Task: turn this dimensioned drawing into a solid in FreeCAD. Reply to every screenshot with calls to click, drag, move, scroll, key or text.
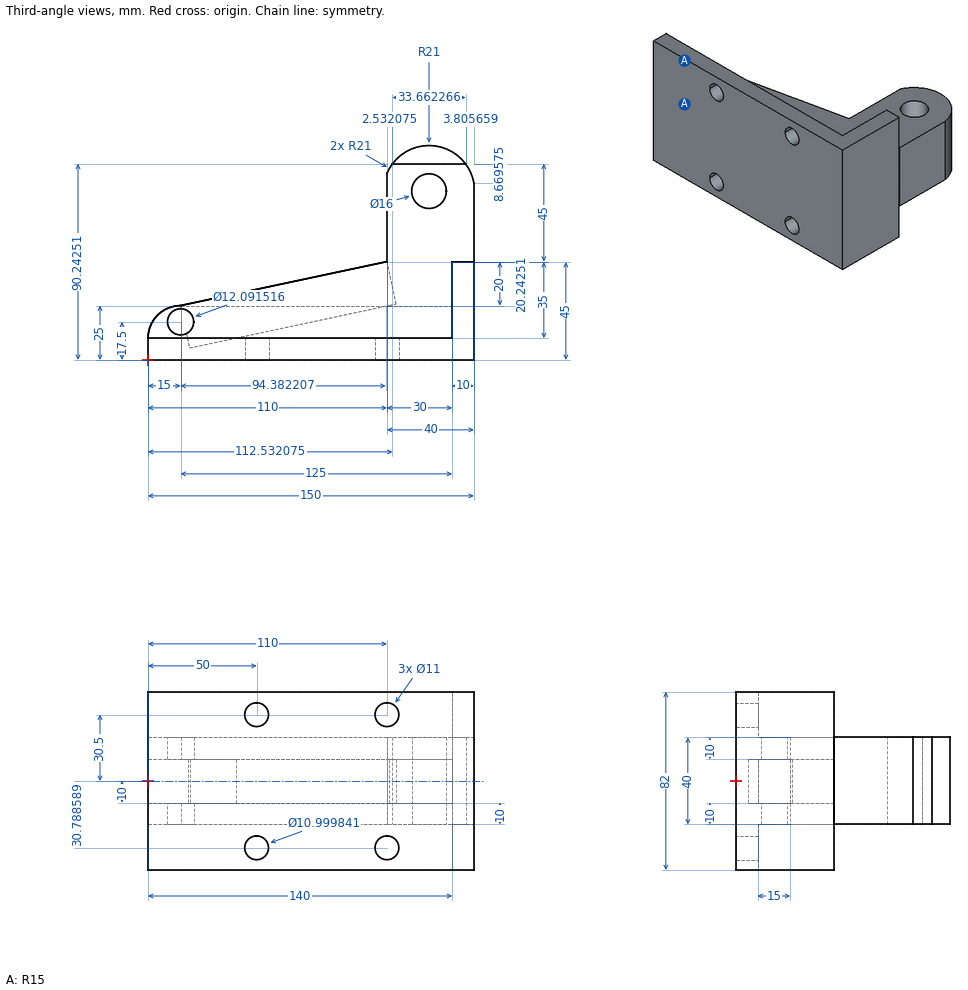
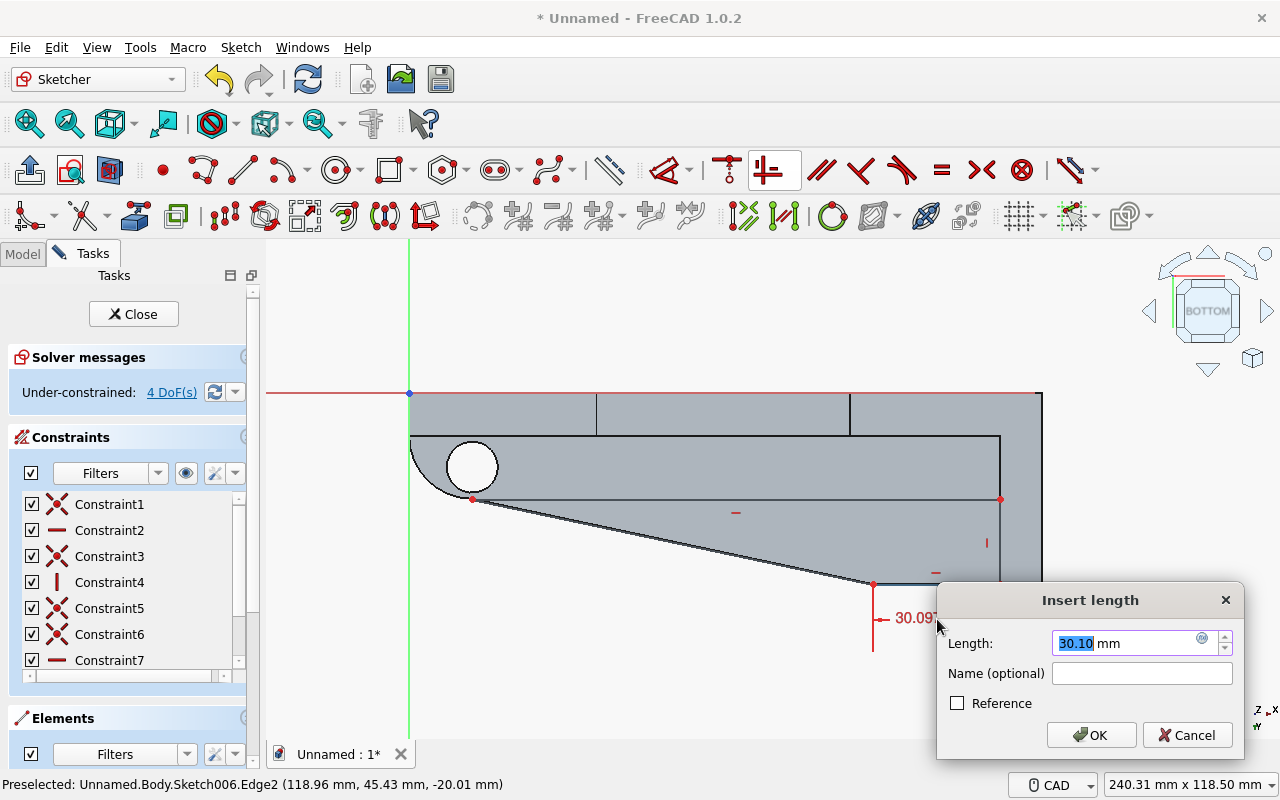
text(30)
key(Return)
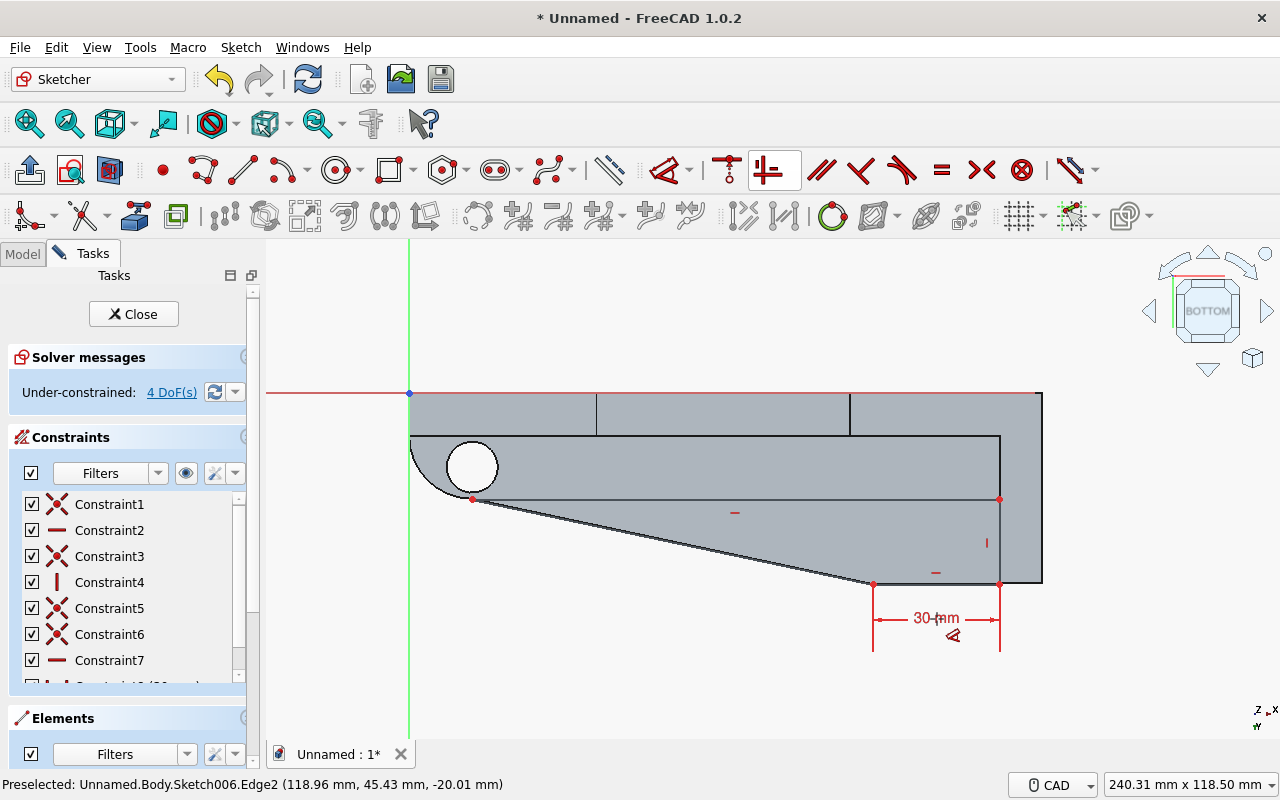
click(841, 500)
click(736, 534)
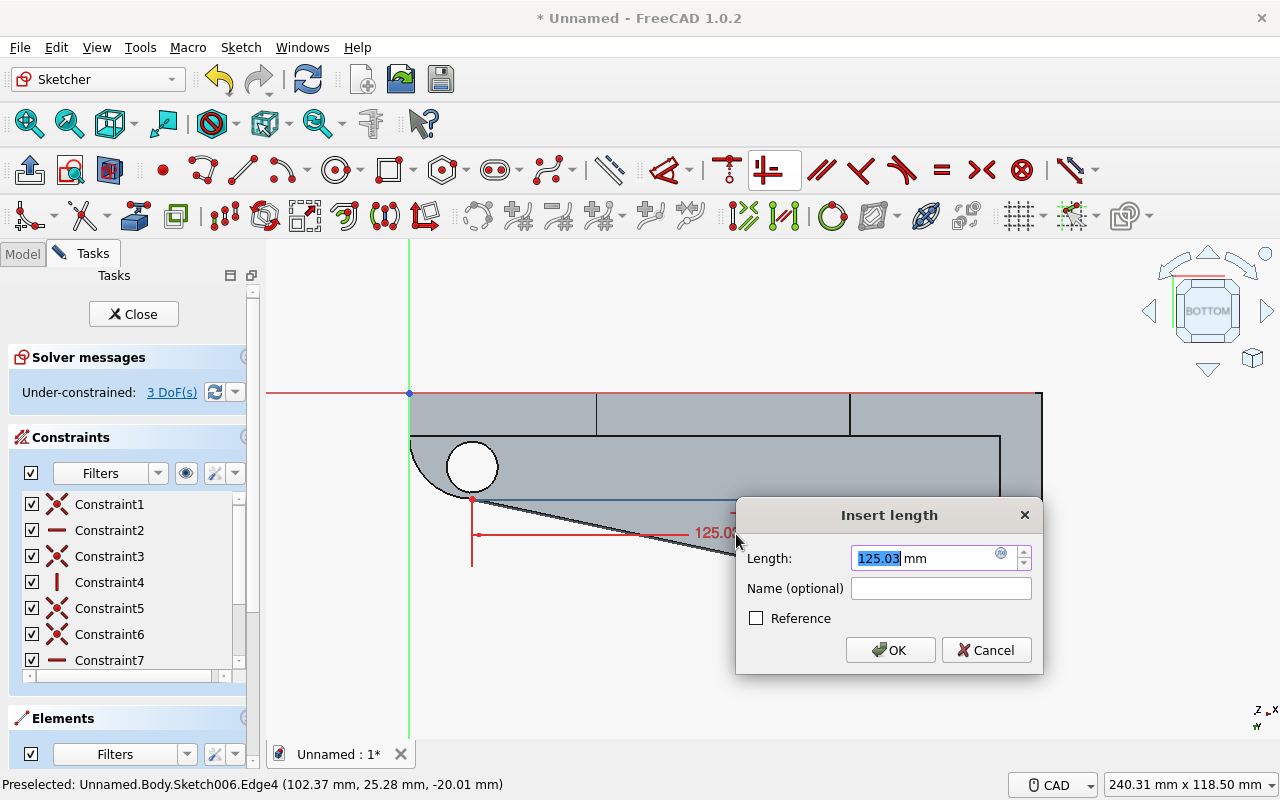
text(125)
key(Return)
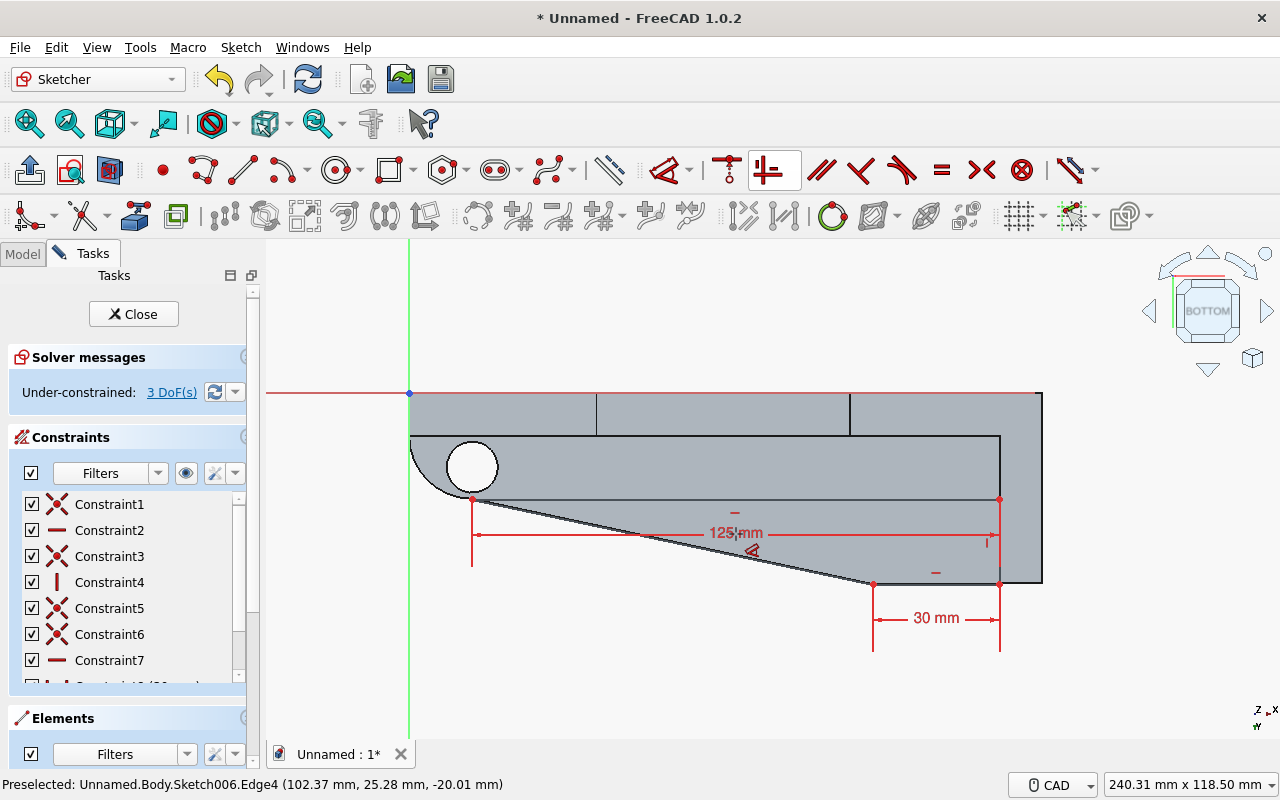
click(472, 500)
click(441, 359)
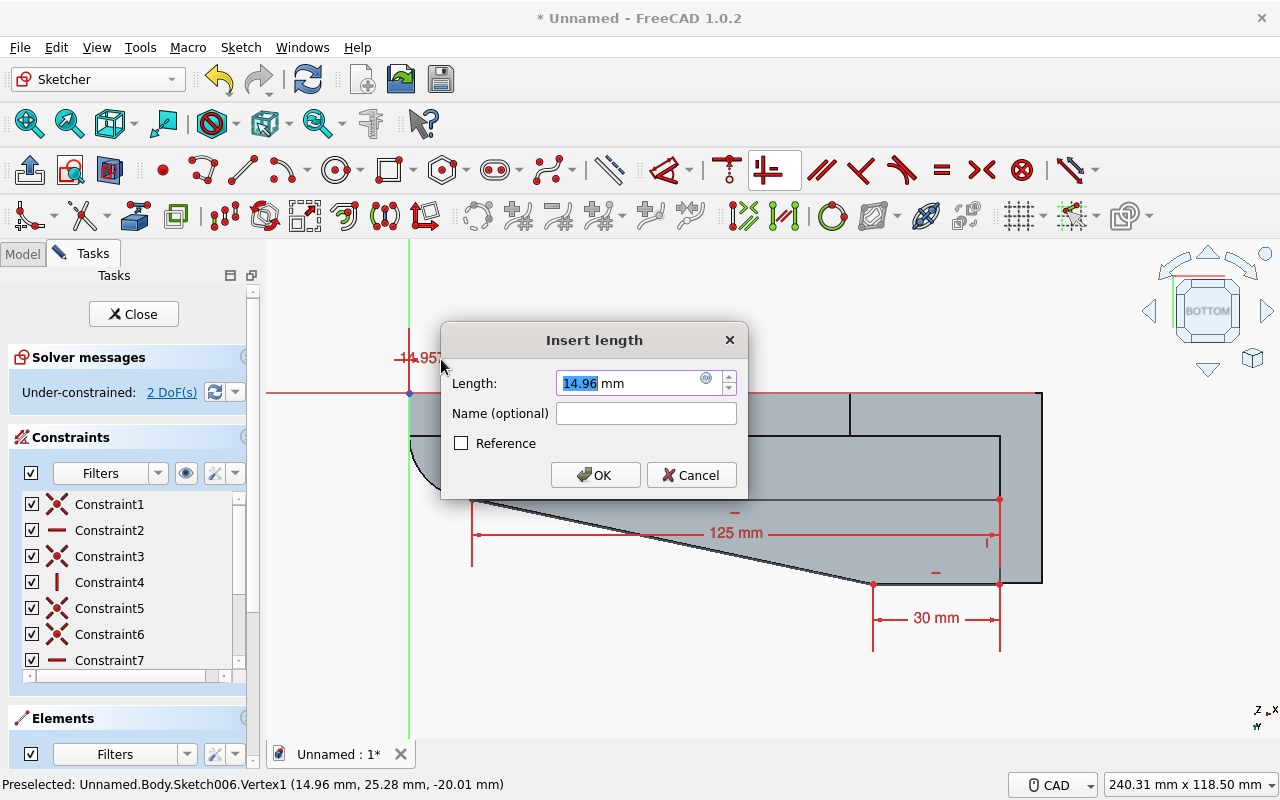
text(15)
key(Return)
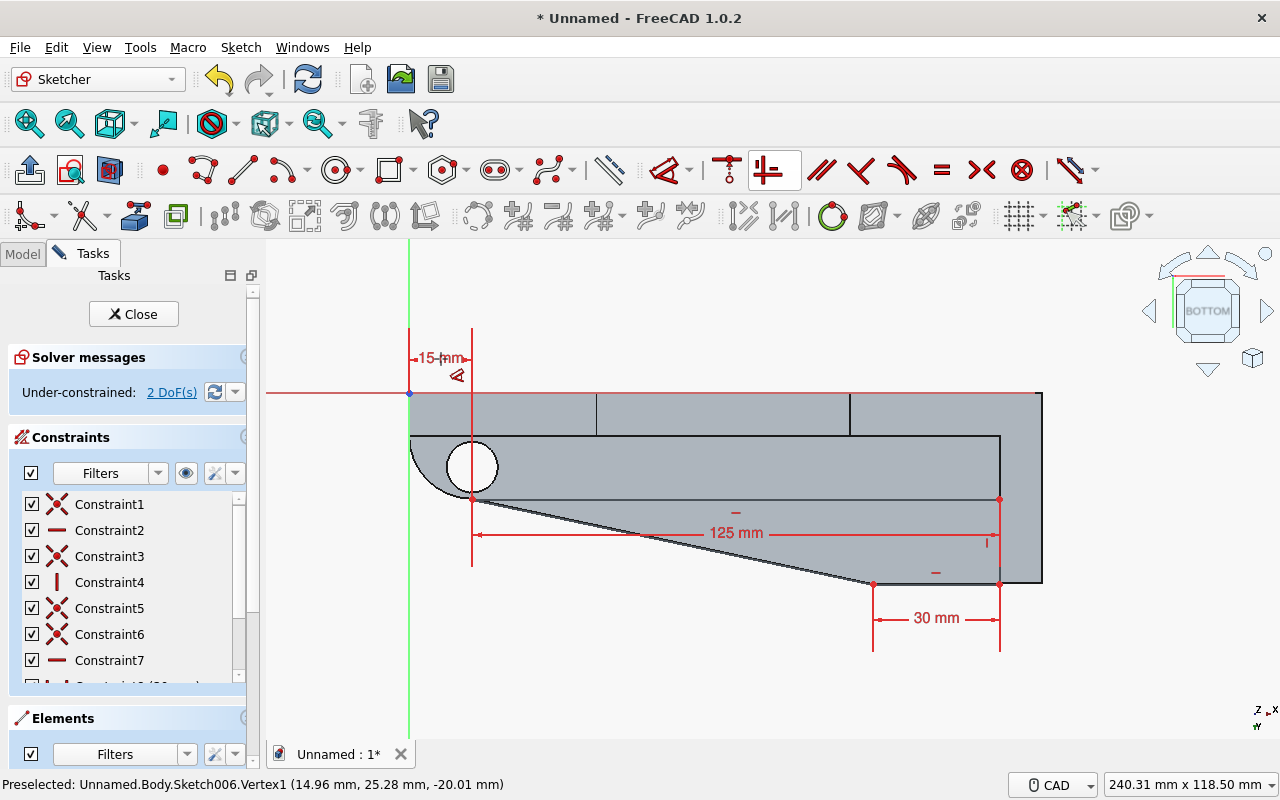
click(472, 500)
click(375, 447)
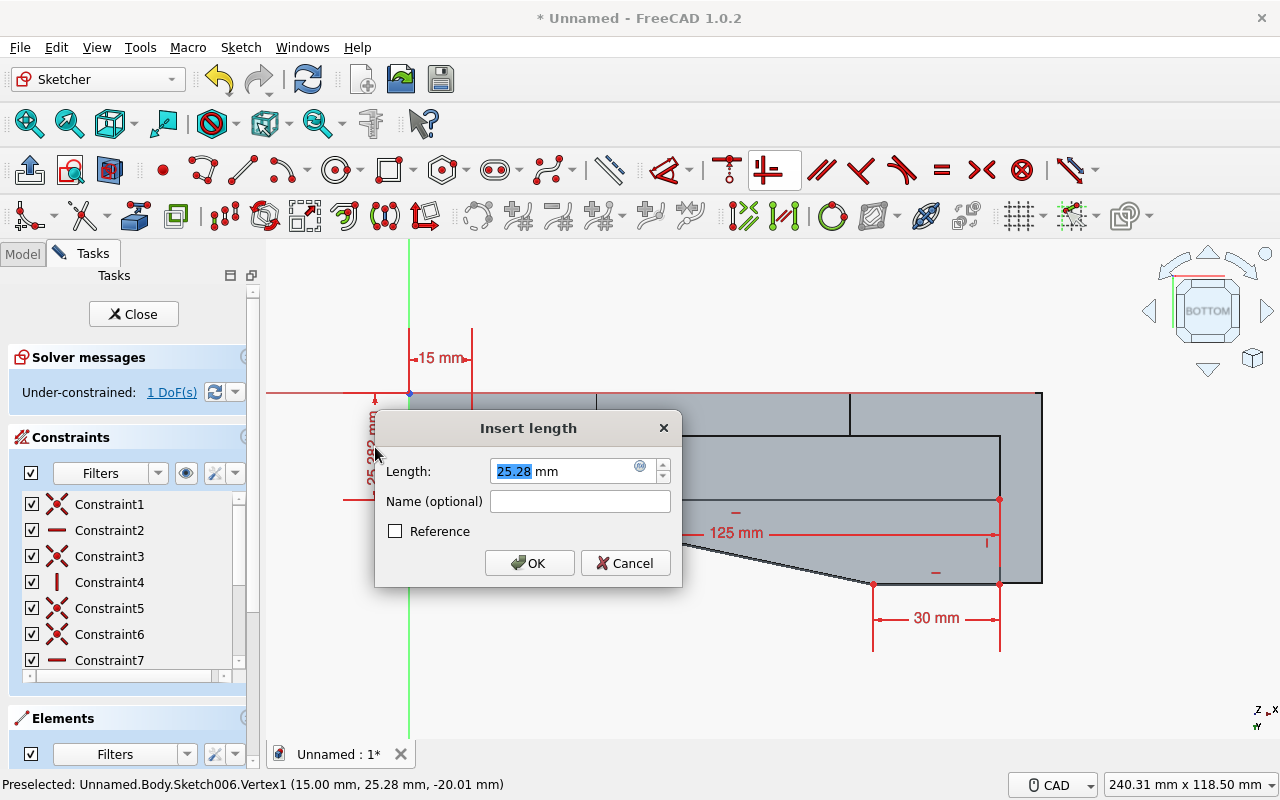
text(25)
key(Return)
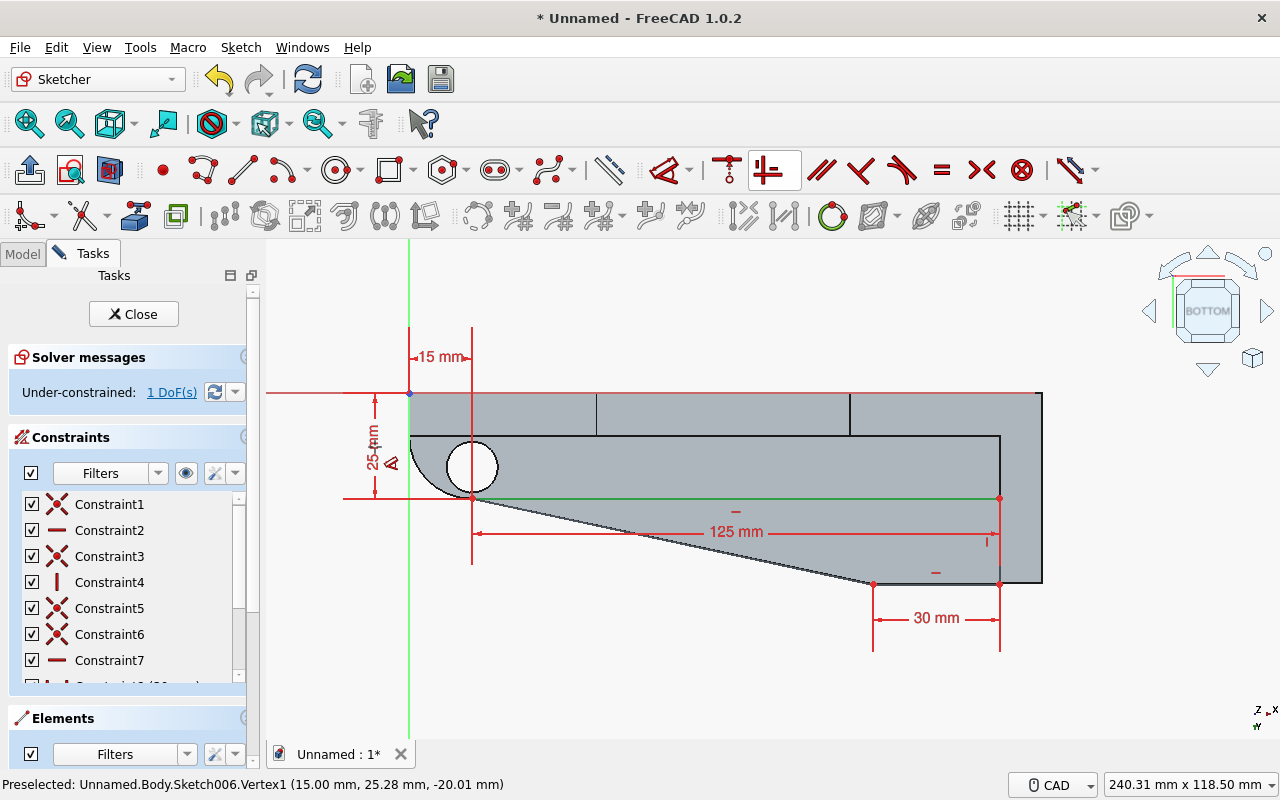
click(1000, 559)
click(1034, 542)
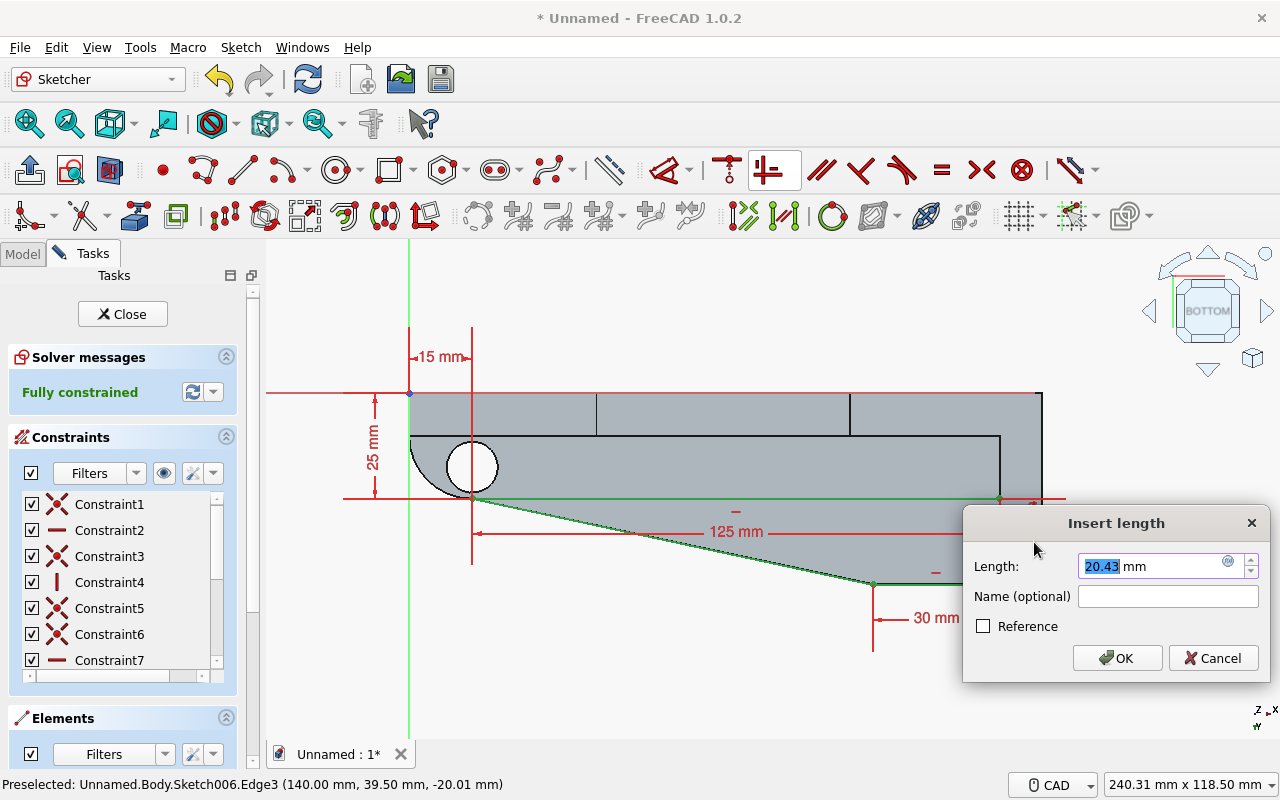
text(20.24251)
key(Return)
key(Escape)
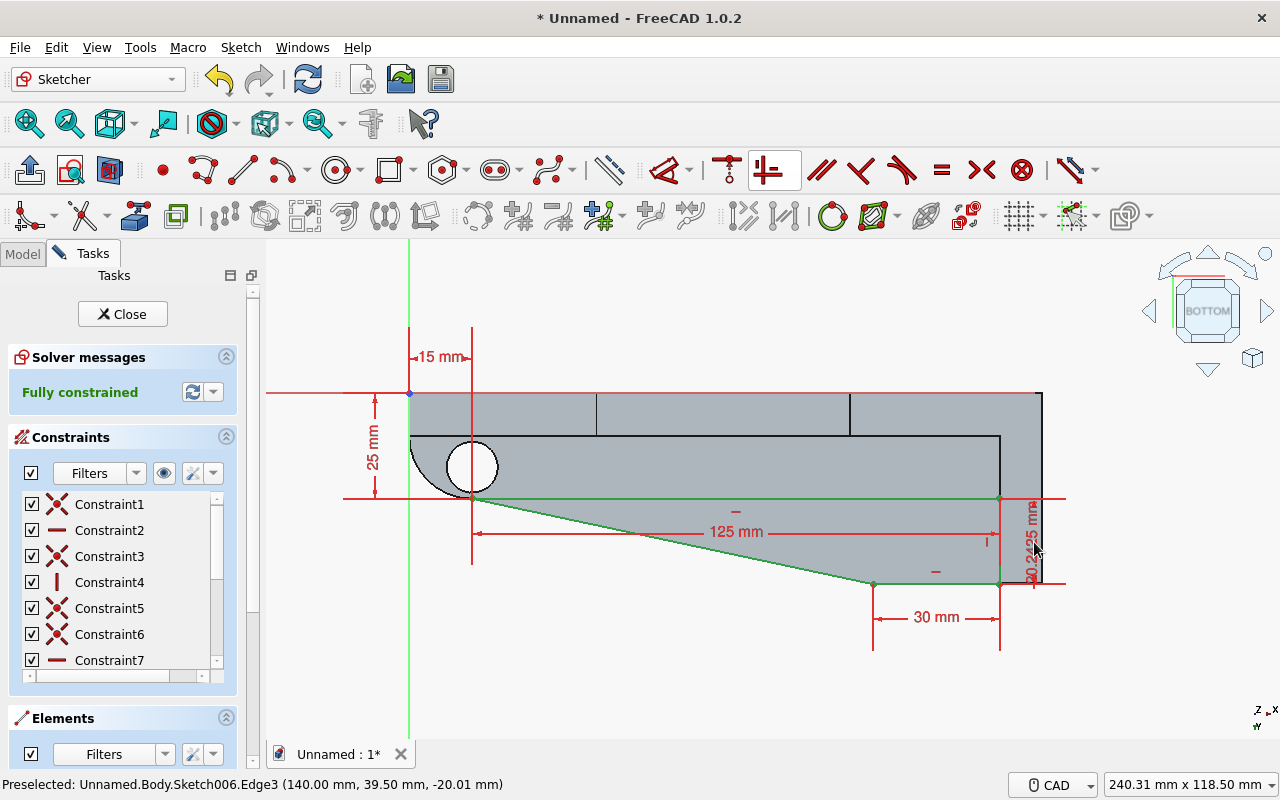
click(123, 314)